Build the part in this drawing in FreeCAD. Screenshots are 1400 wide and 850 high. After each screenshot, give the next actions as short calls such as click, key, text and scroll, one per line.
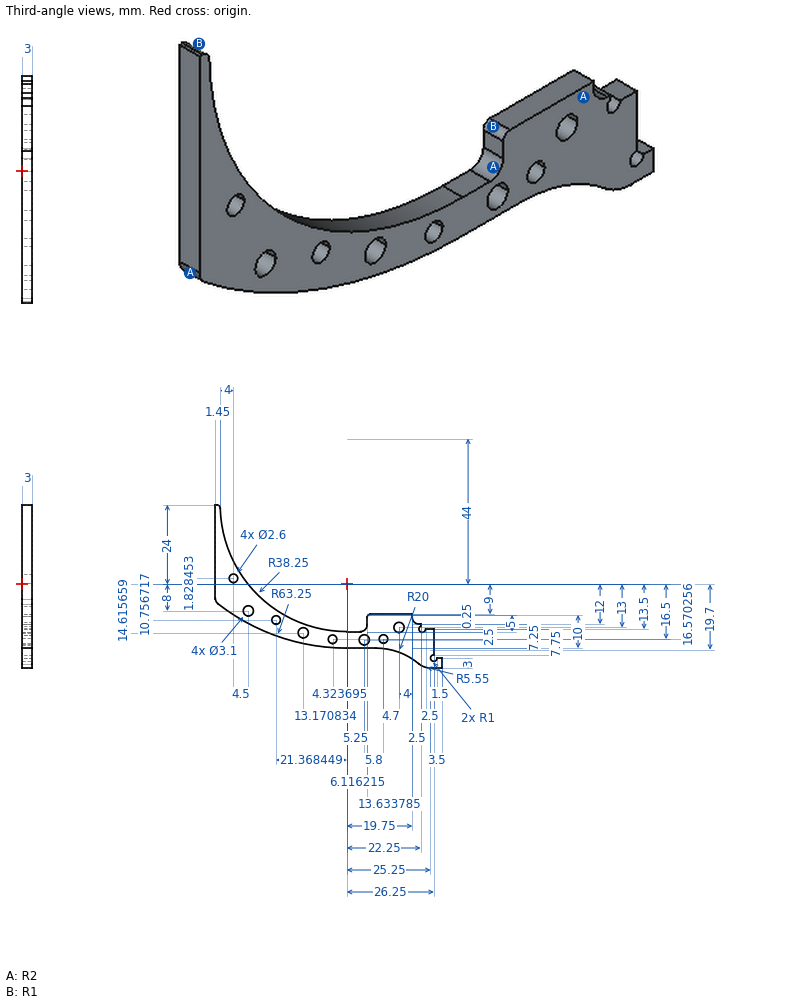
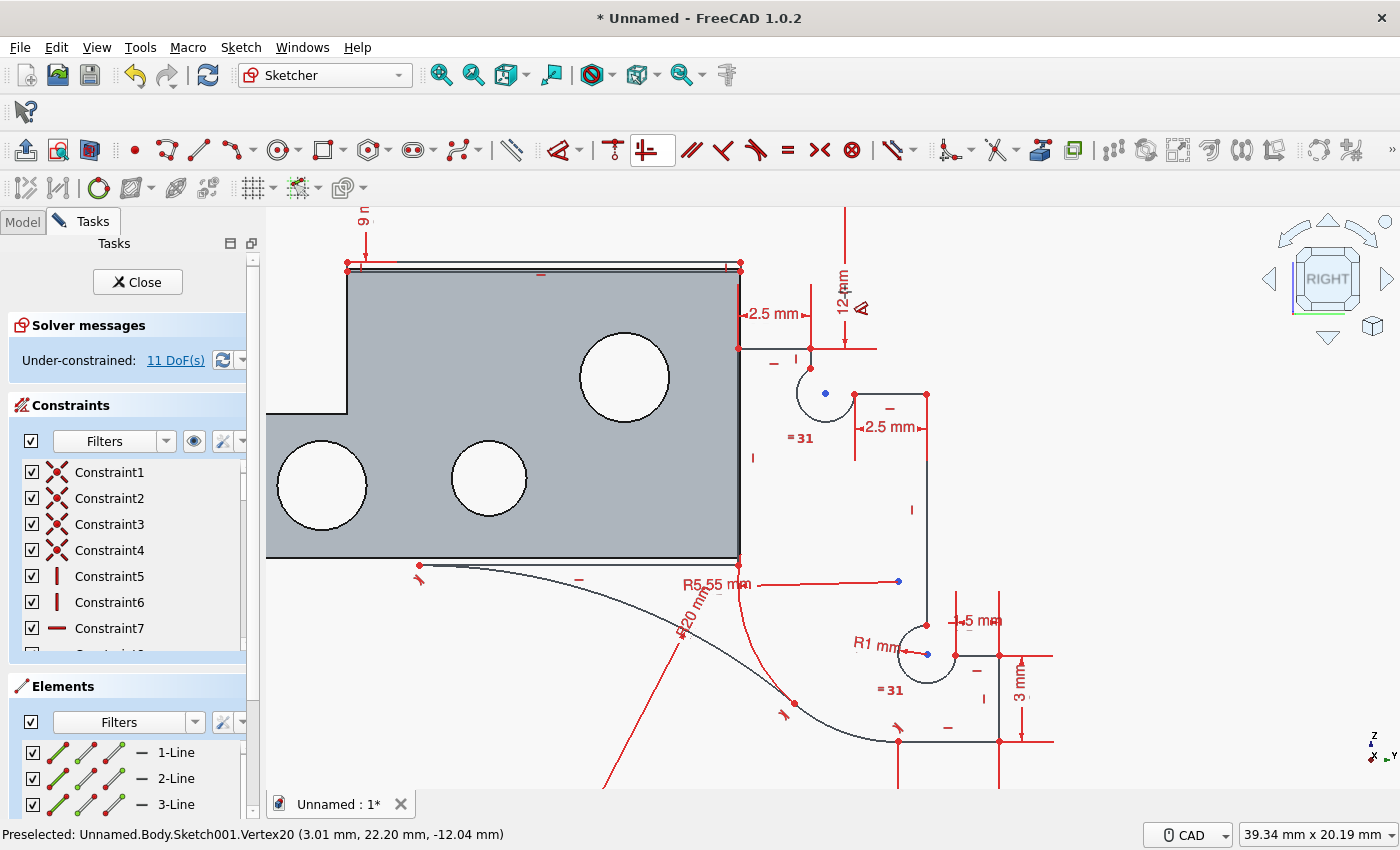
scroll(347, 267, up, 9)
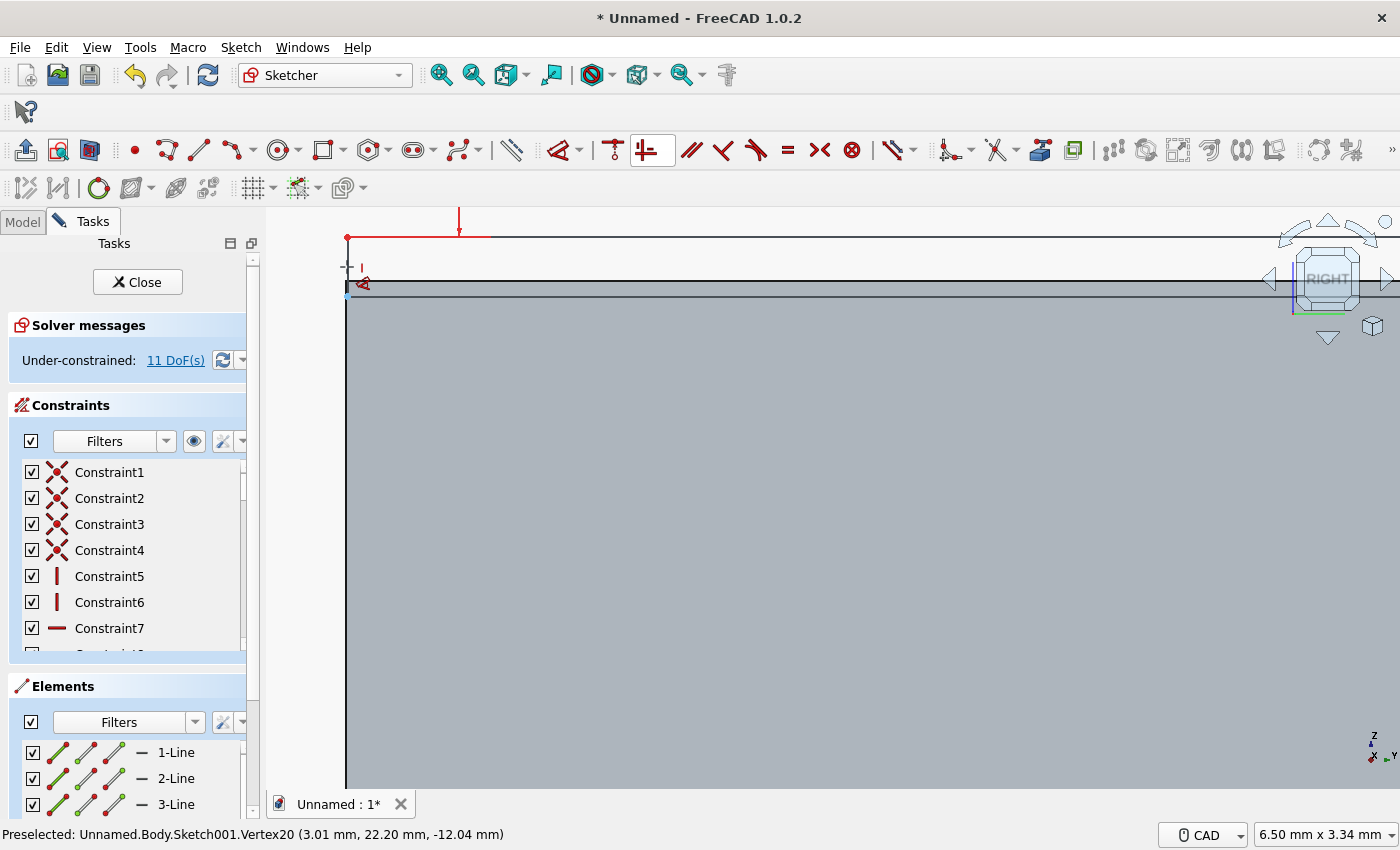
click(348, 267)
click(314, 267)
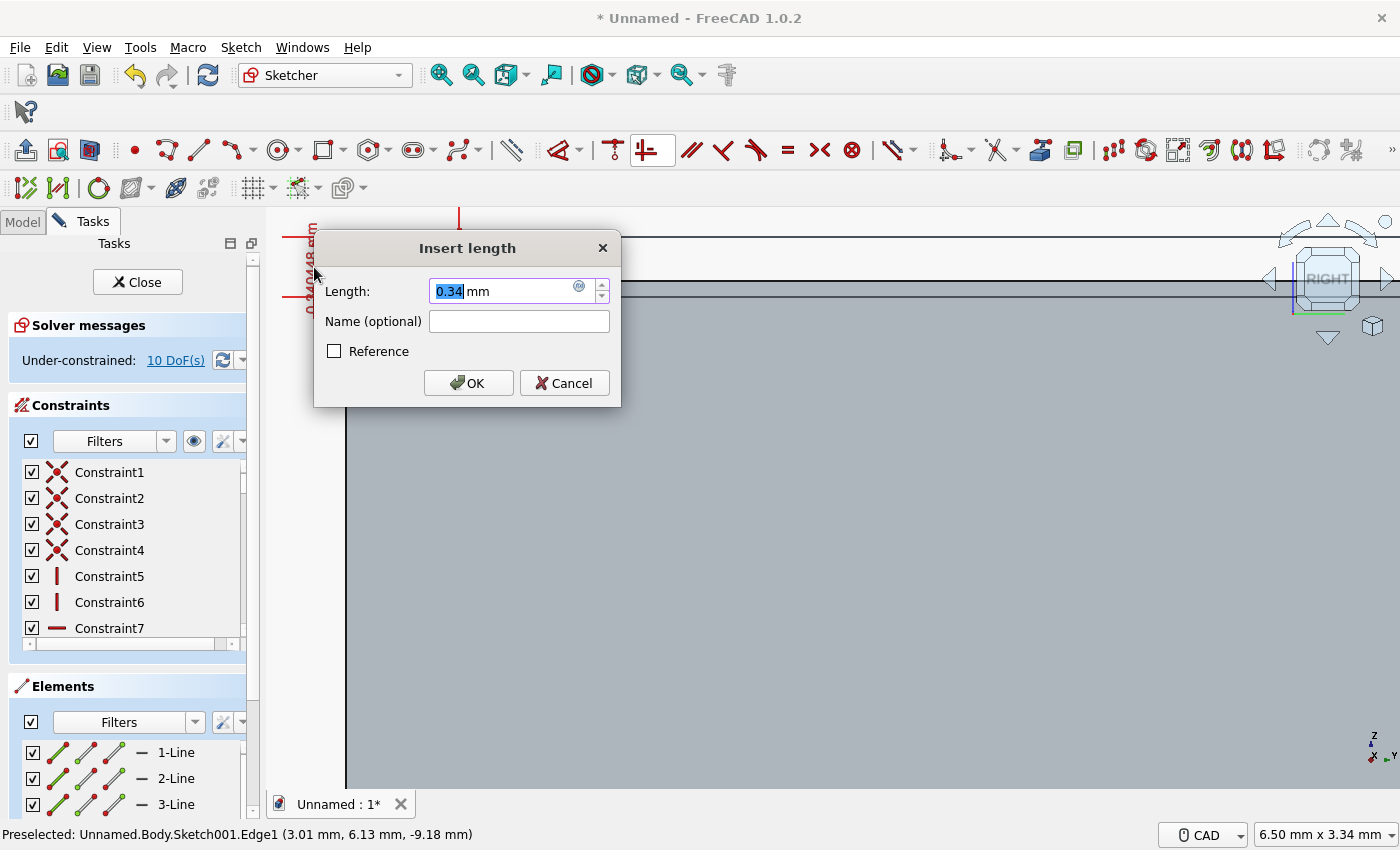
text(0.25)
key(Return)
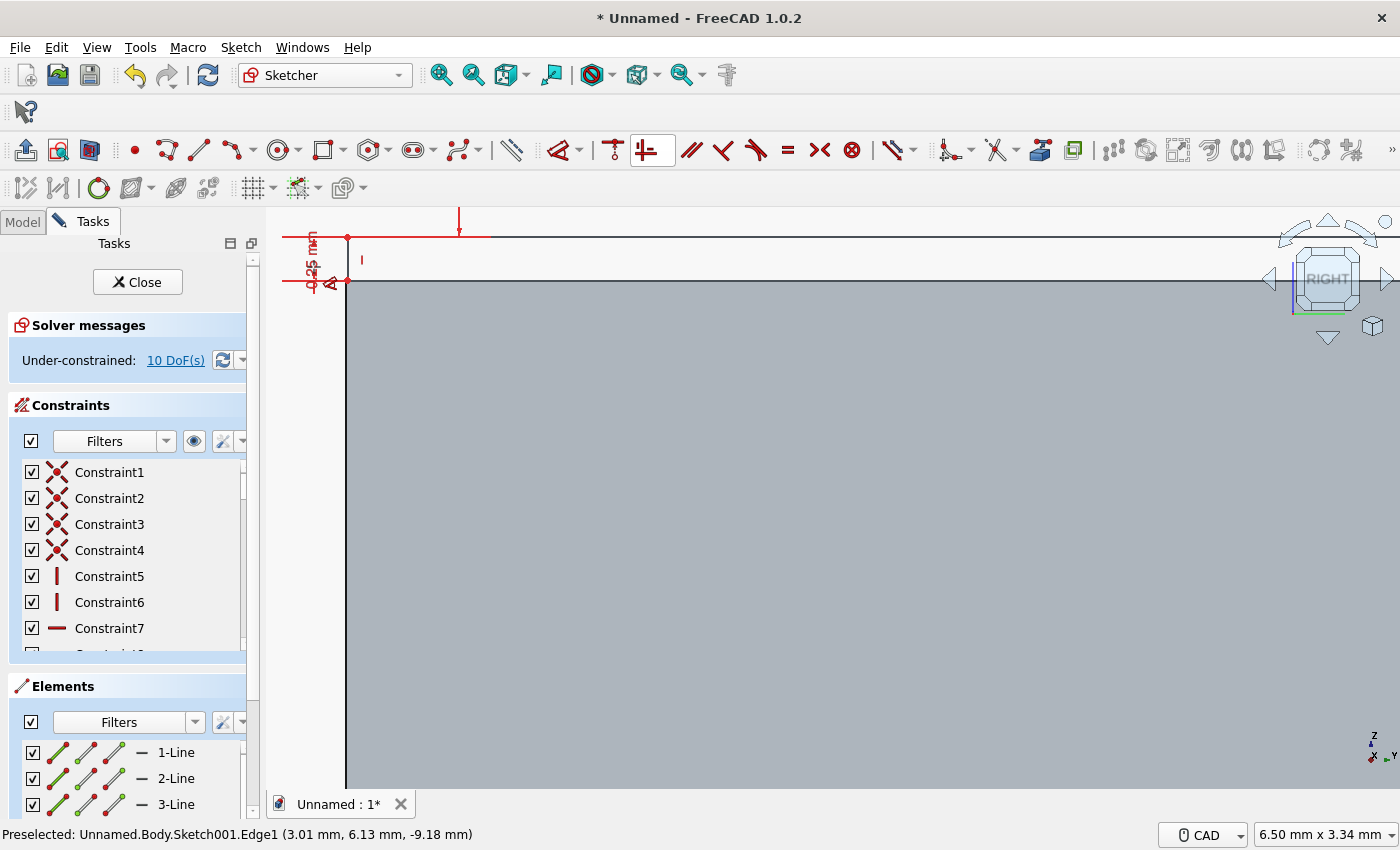
scroll(663, 461, down, 12)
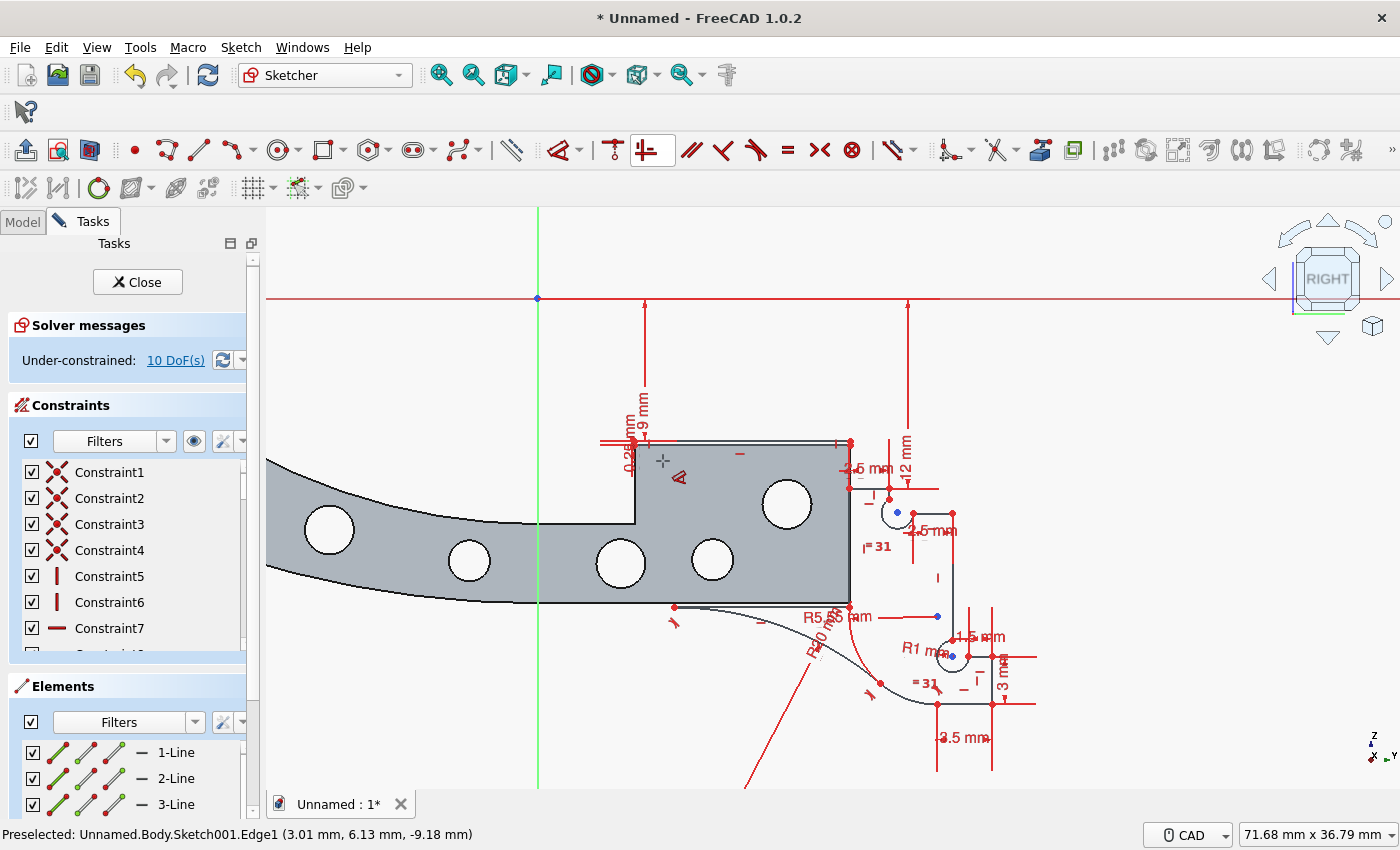
click(953, 602)
click(987, 577)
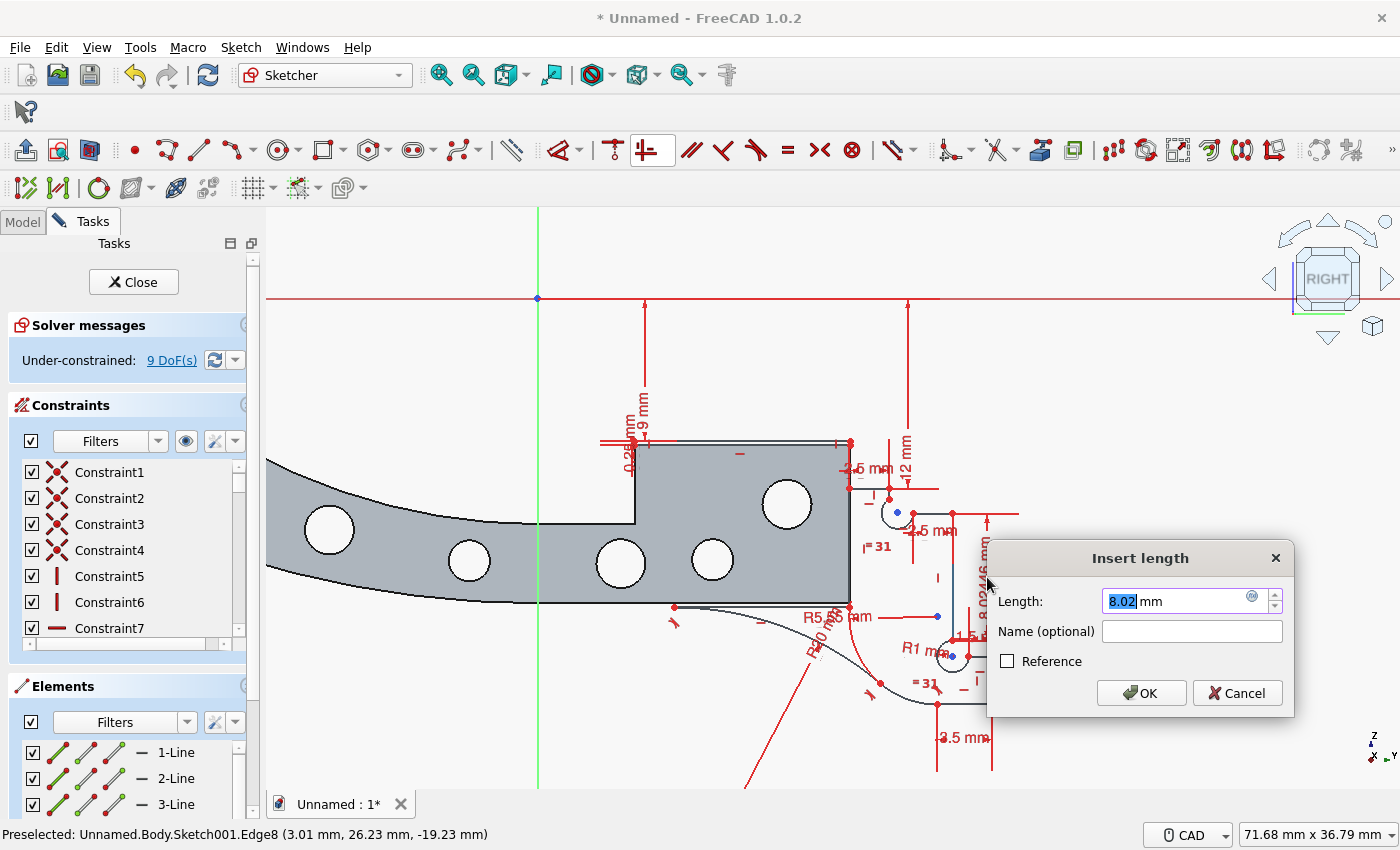
text(7.75)
key(Return)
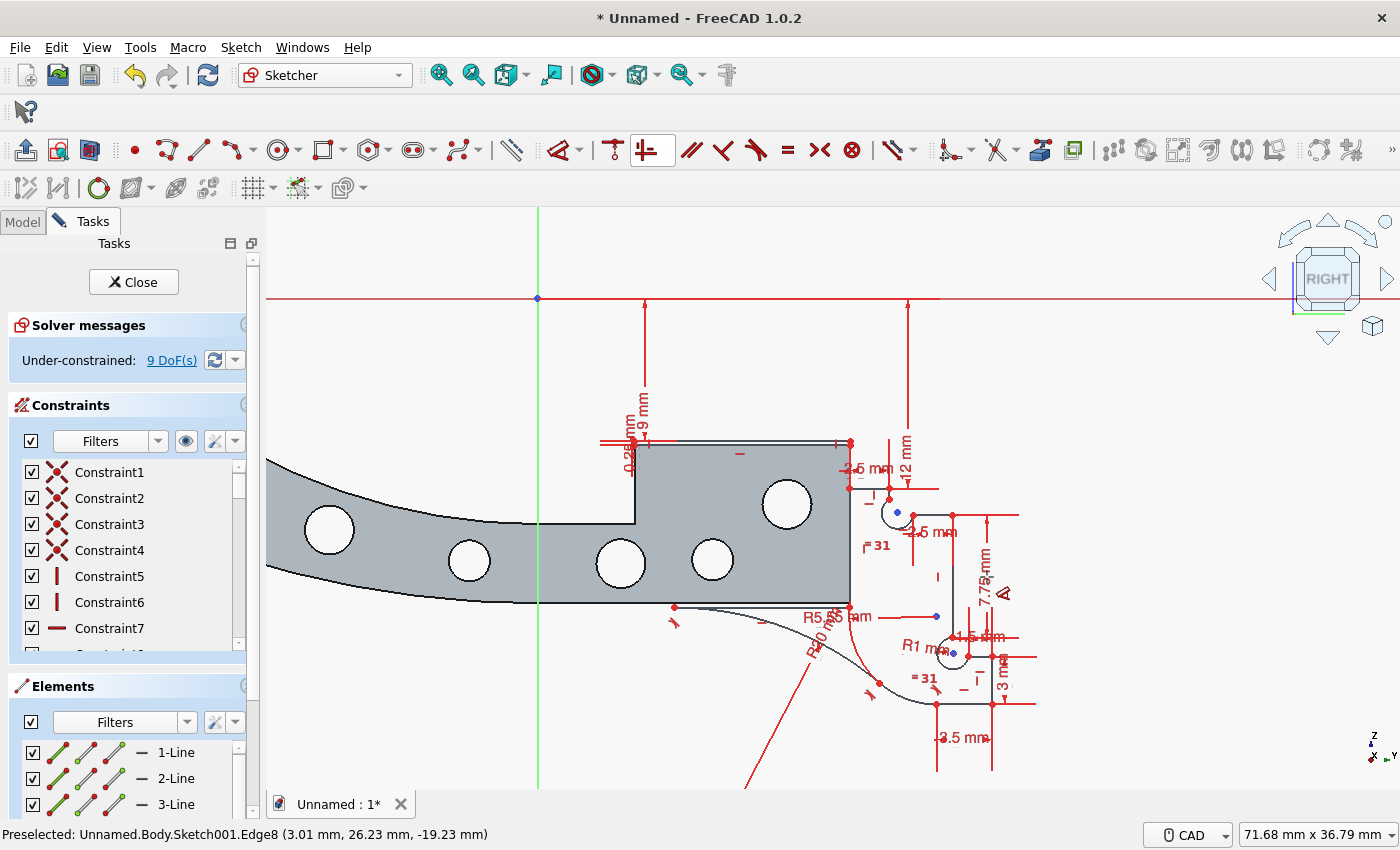
click(850, 524)
click(884, 575)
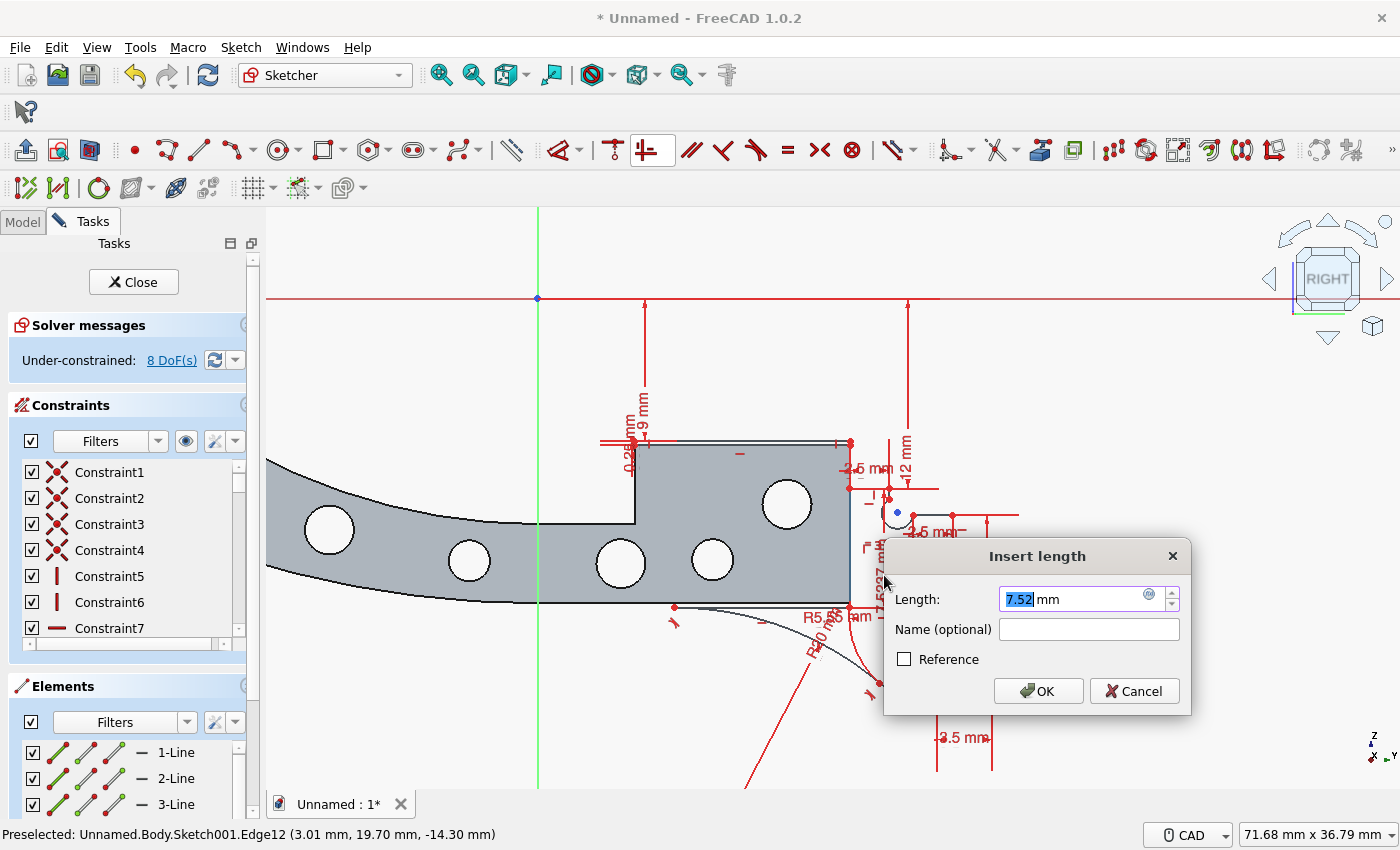
text(7.25)
key(Return)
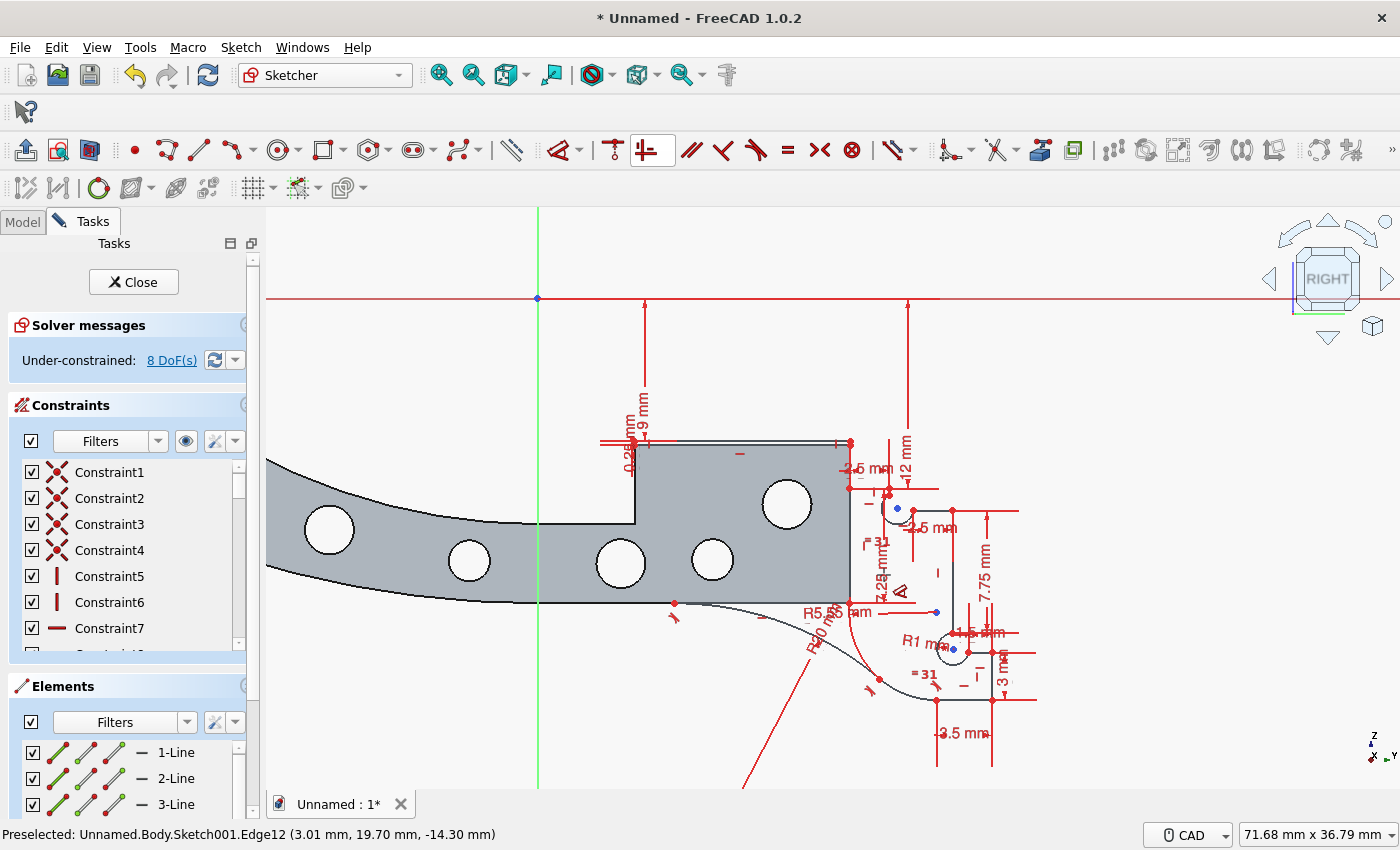
click(953, 511)
click(504, 405)